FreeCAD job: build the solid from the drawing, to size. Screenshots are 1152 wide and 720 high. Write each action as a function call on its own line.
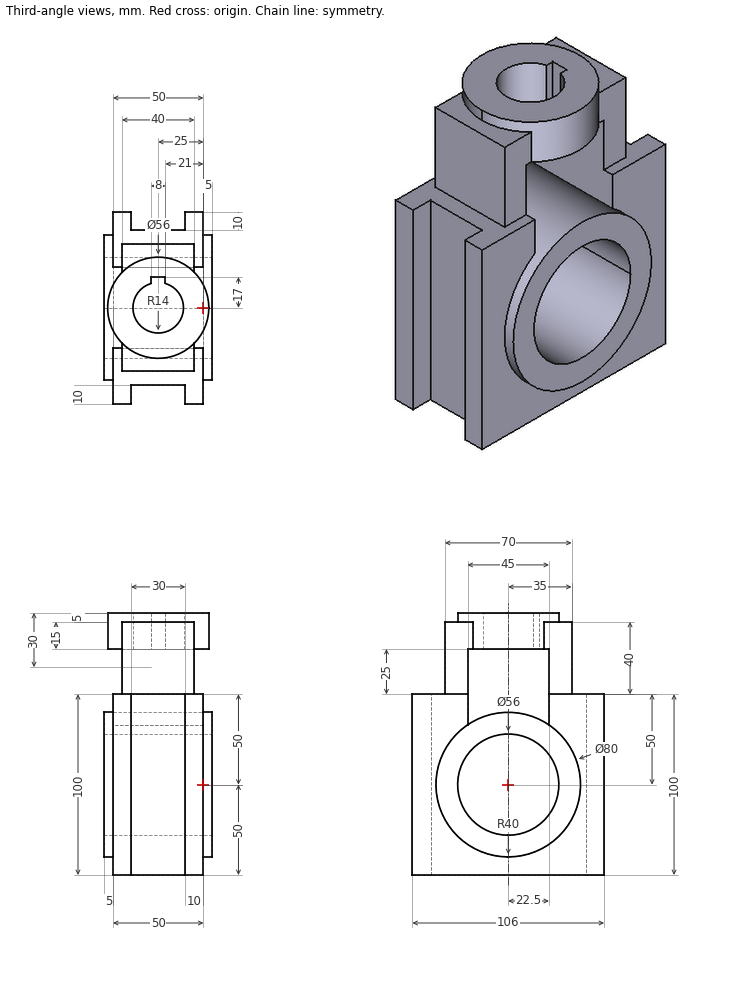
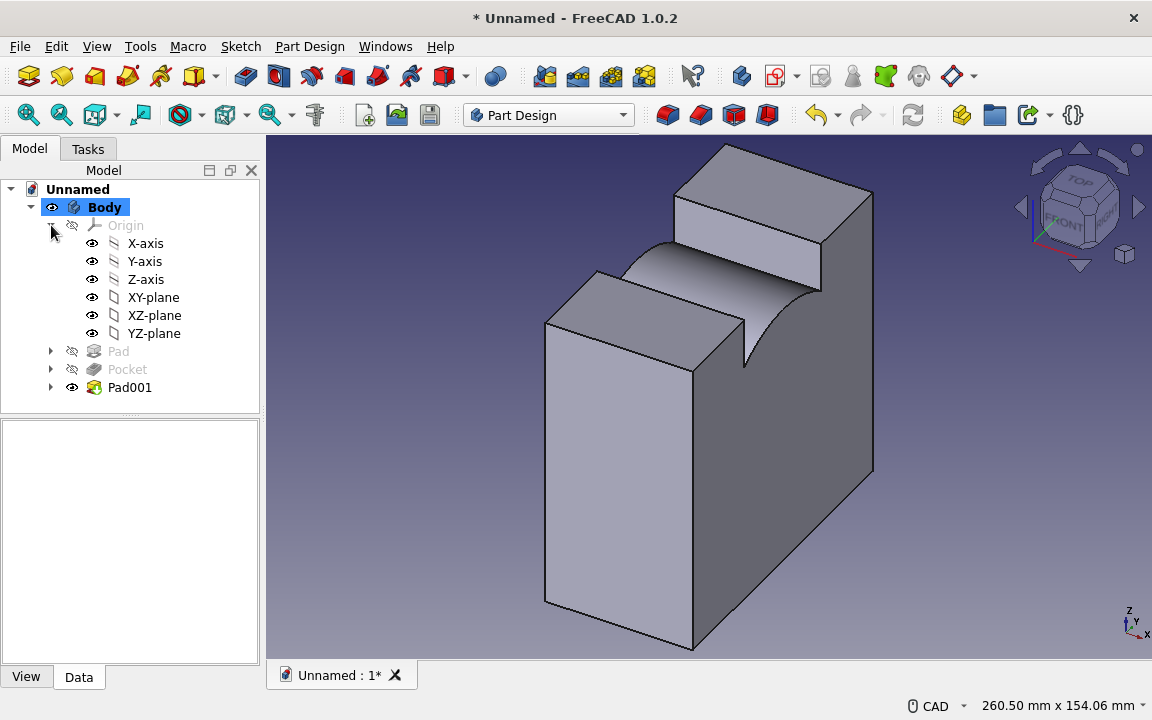
click(137, 333)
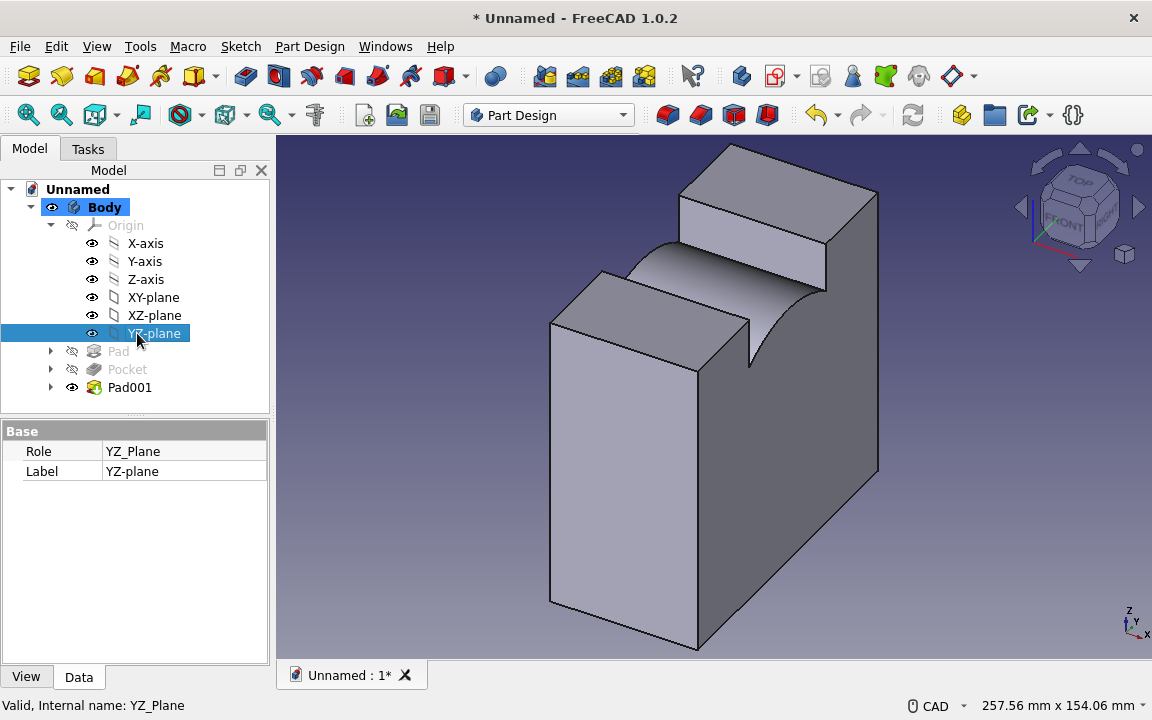
click(952, 76)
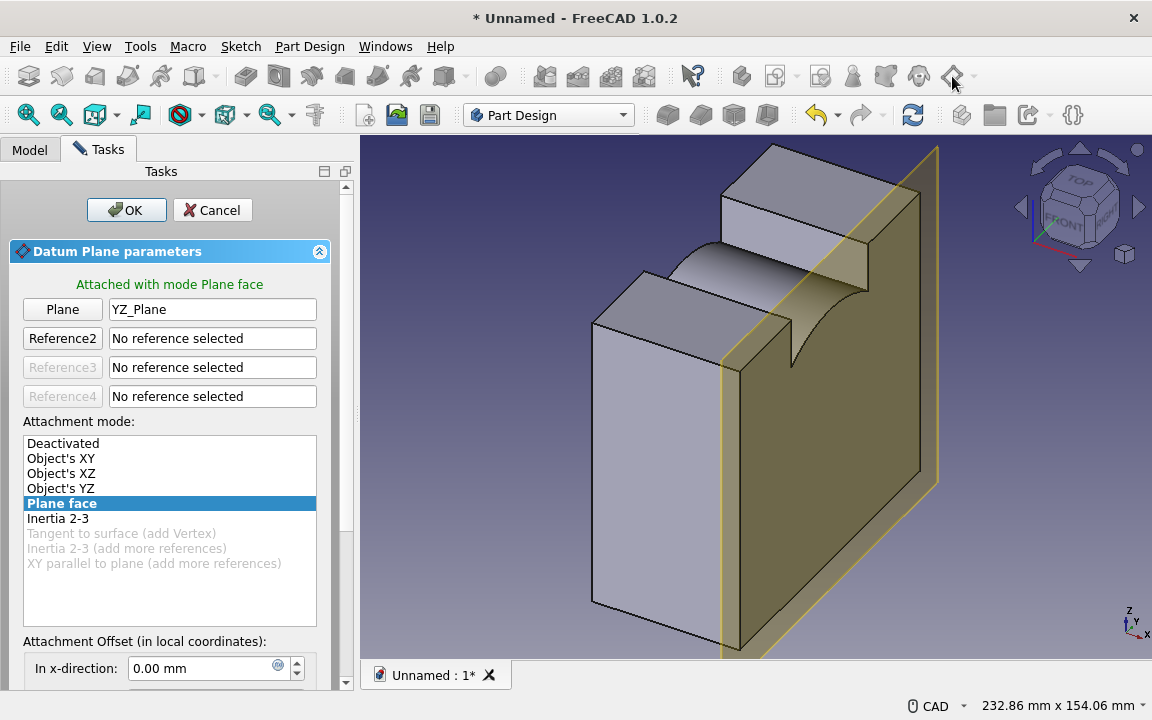
scroll(346, 436, down, 2)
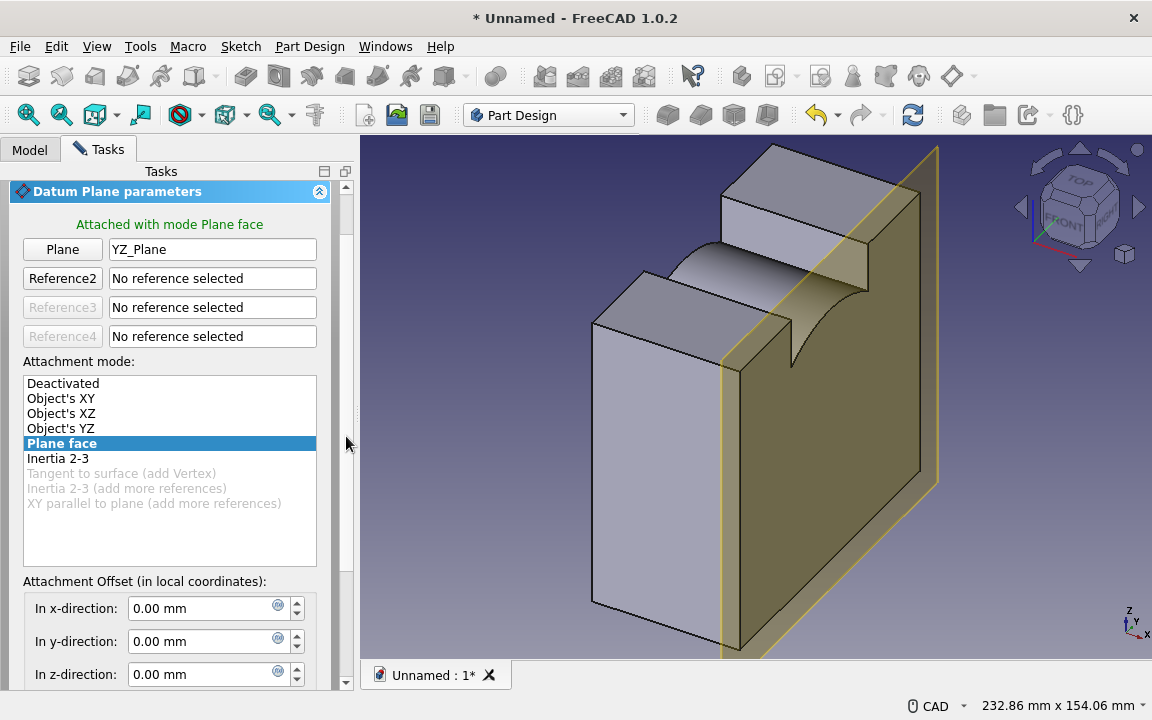
triple_click(210, 614)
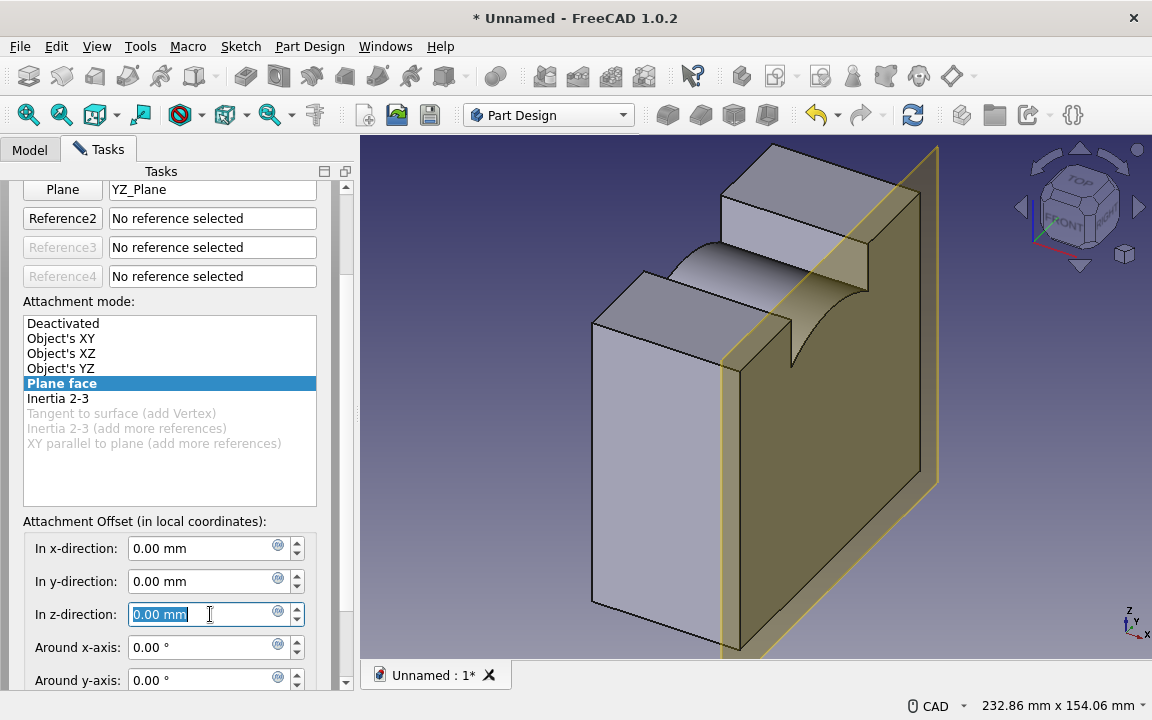
text(5)
key(Tab)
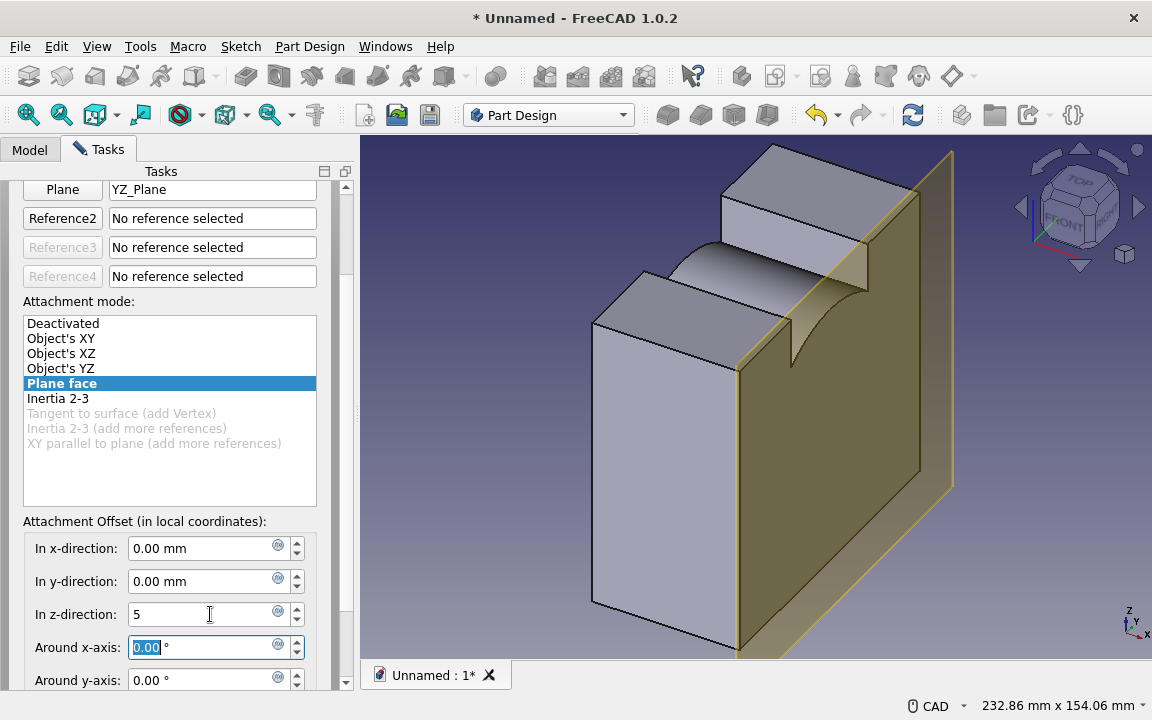
scroll(346, 436, up, 3)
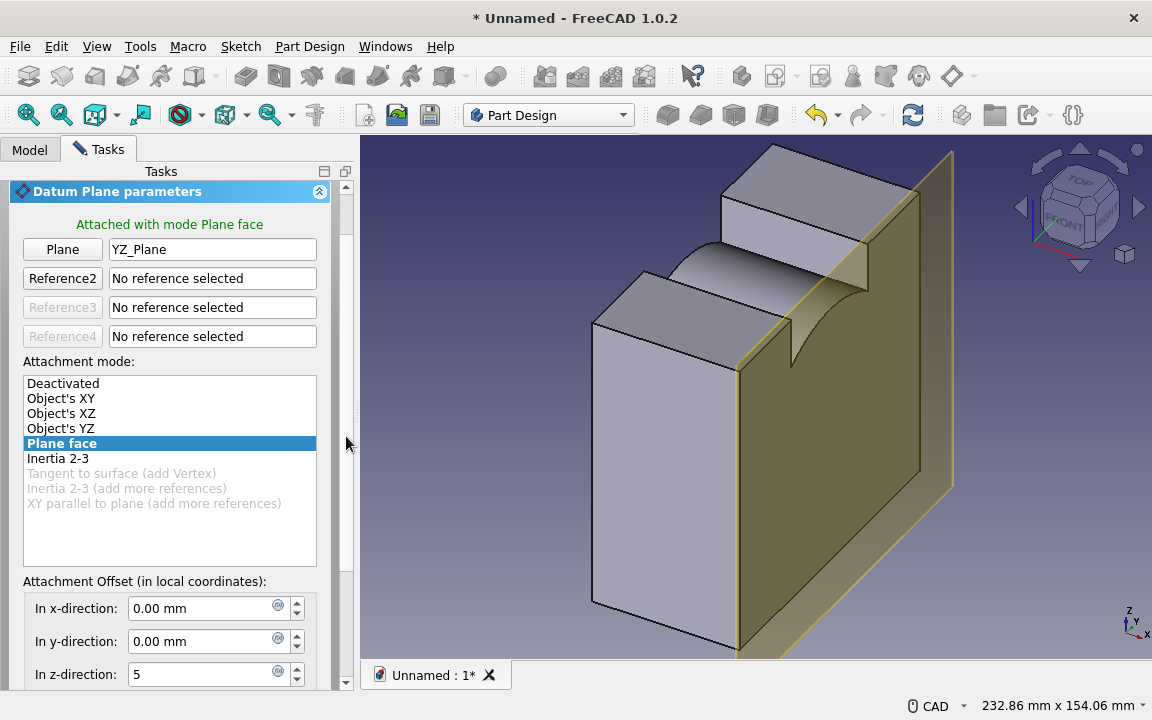
click(127, 210)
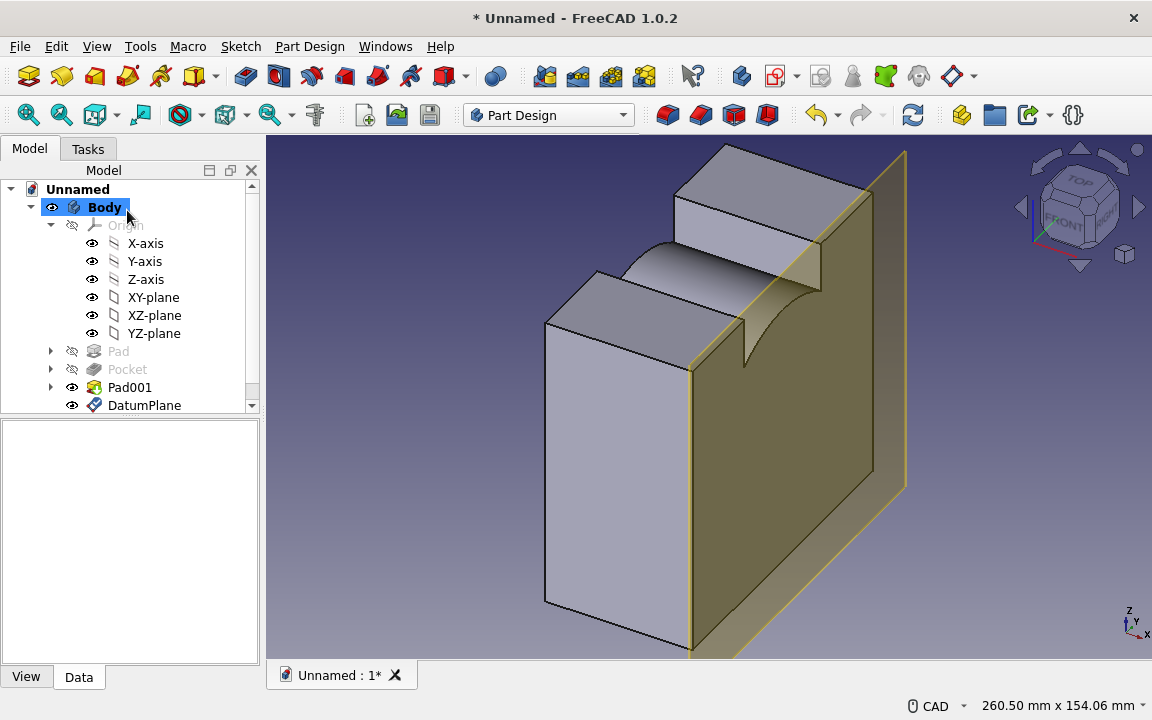
click(117, 405)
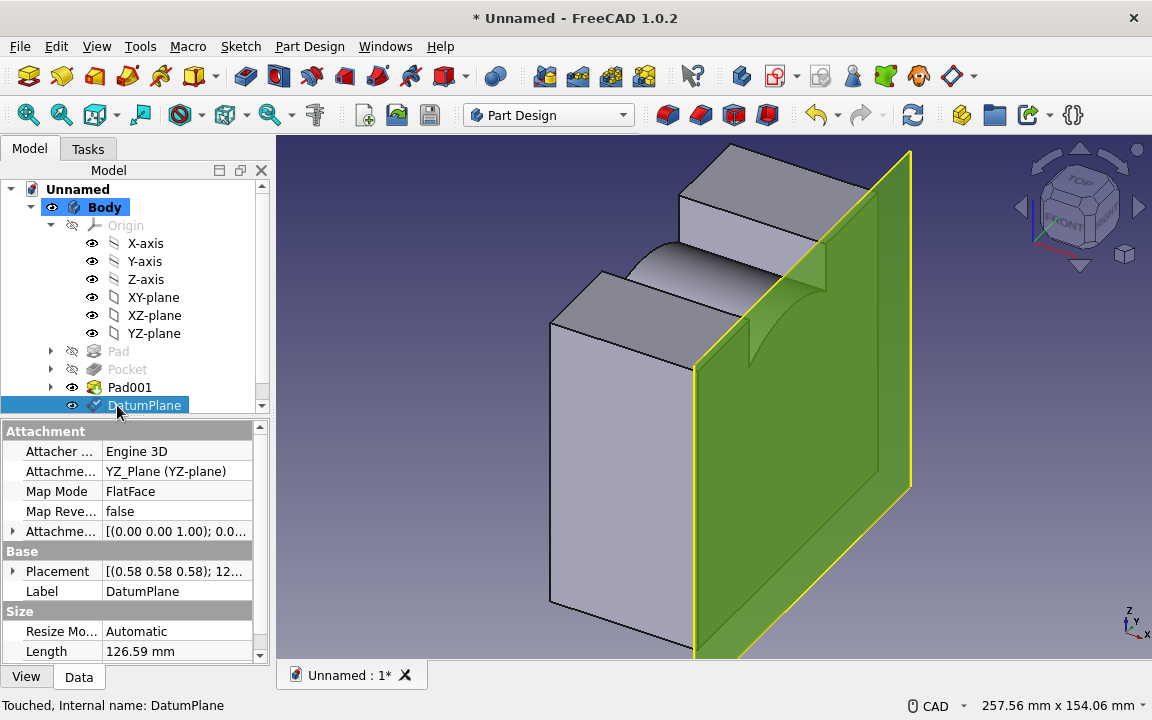
click(774, 76)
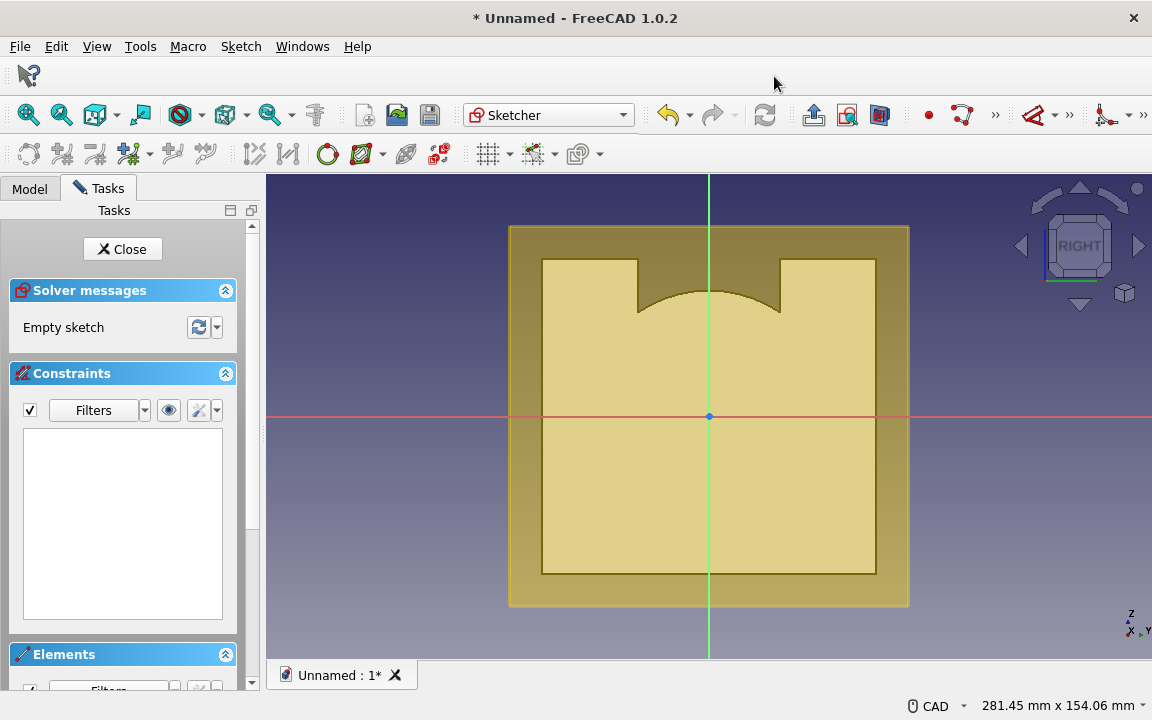
key(g)
key(c)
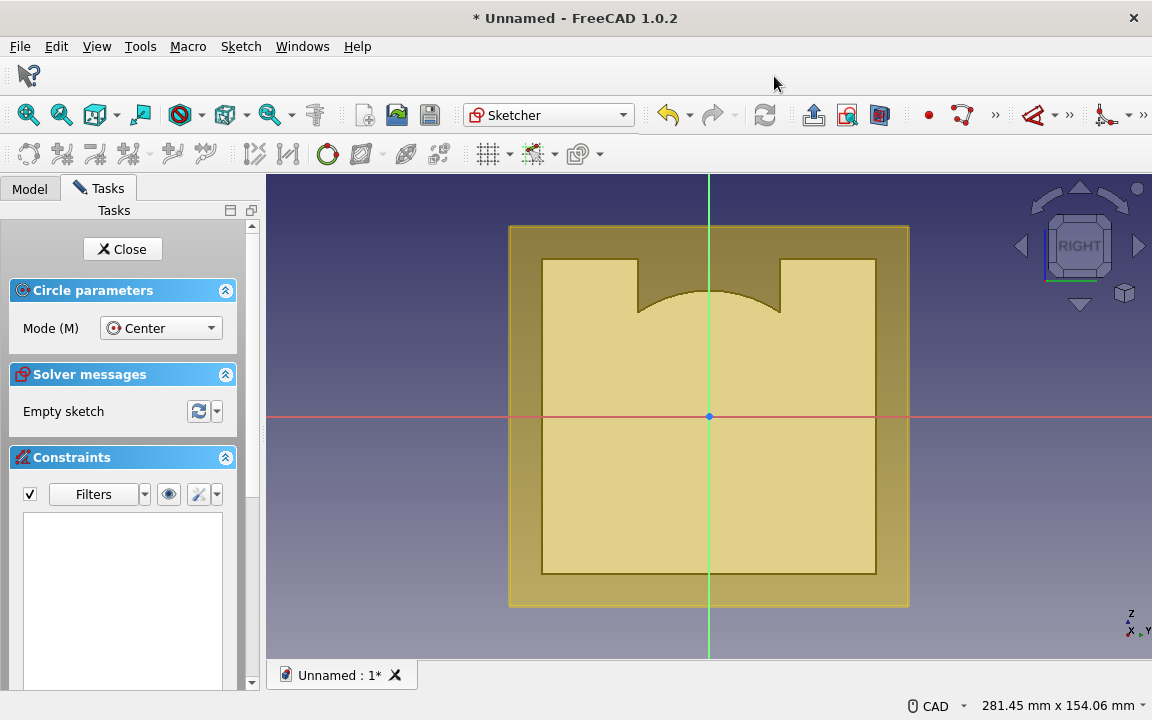
click(709, 416)
move(798, 327)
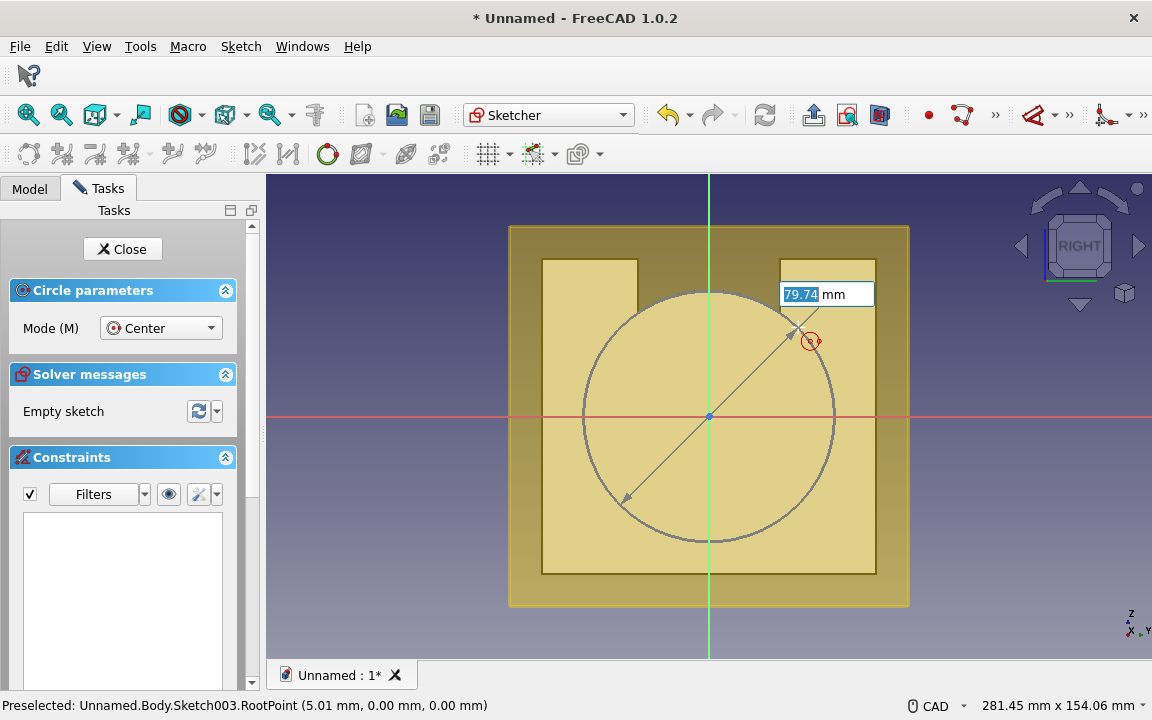
text(80)
key(Return)
key(Escape)